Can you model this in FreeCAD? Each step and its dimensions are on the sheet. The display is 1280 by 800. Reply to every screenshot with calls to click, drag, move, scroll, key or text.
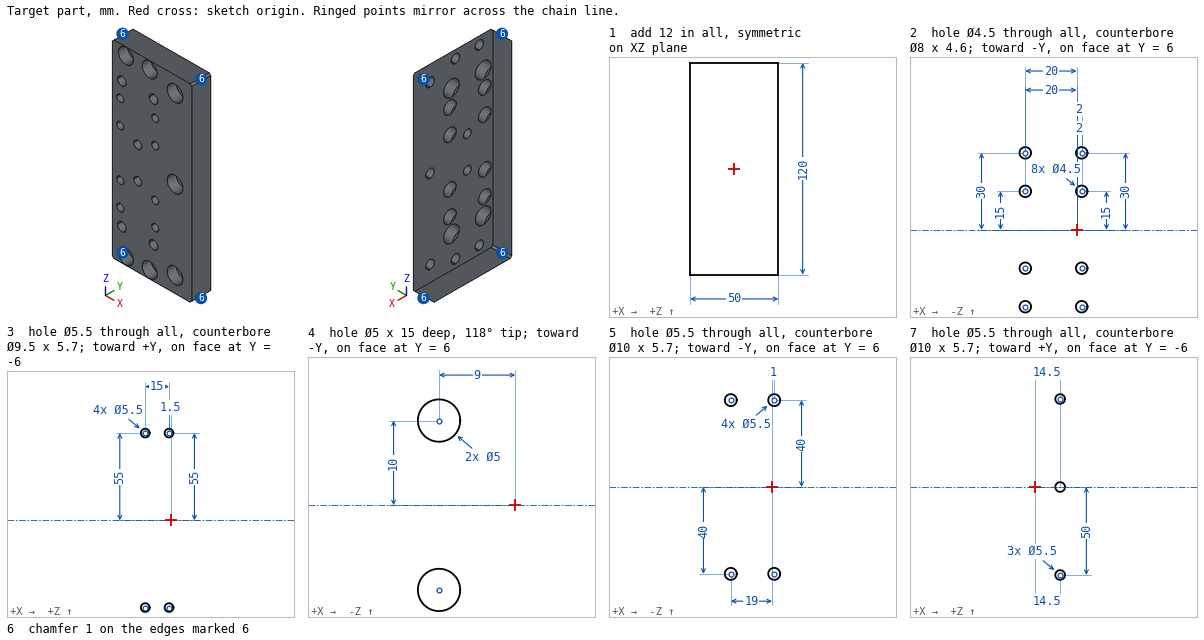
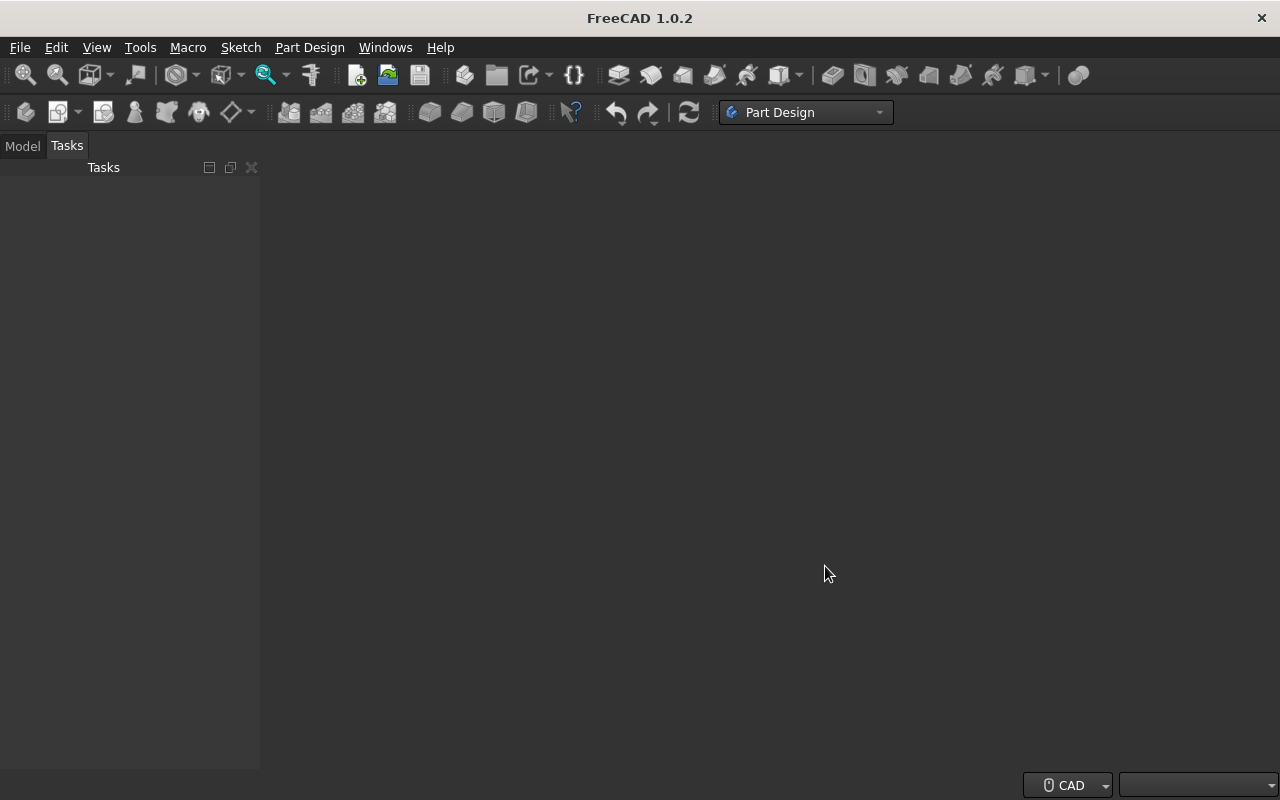
click(356, 76)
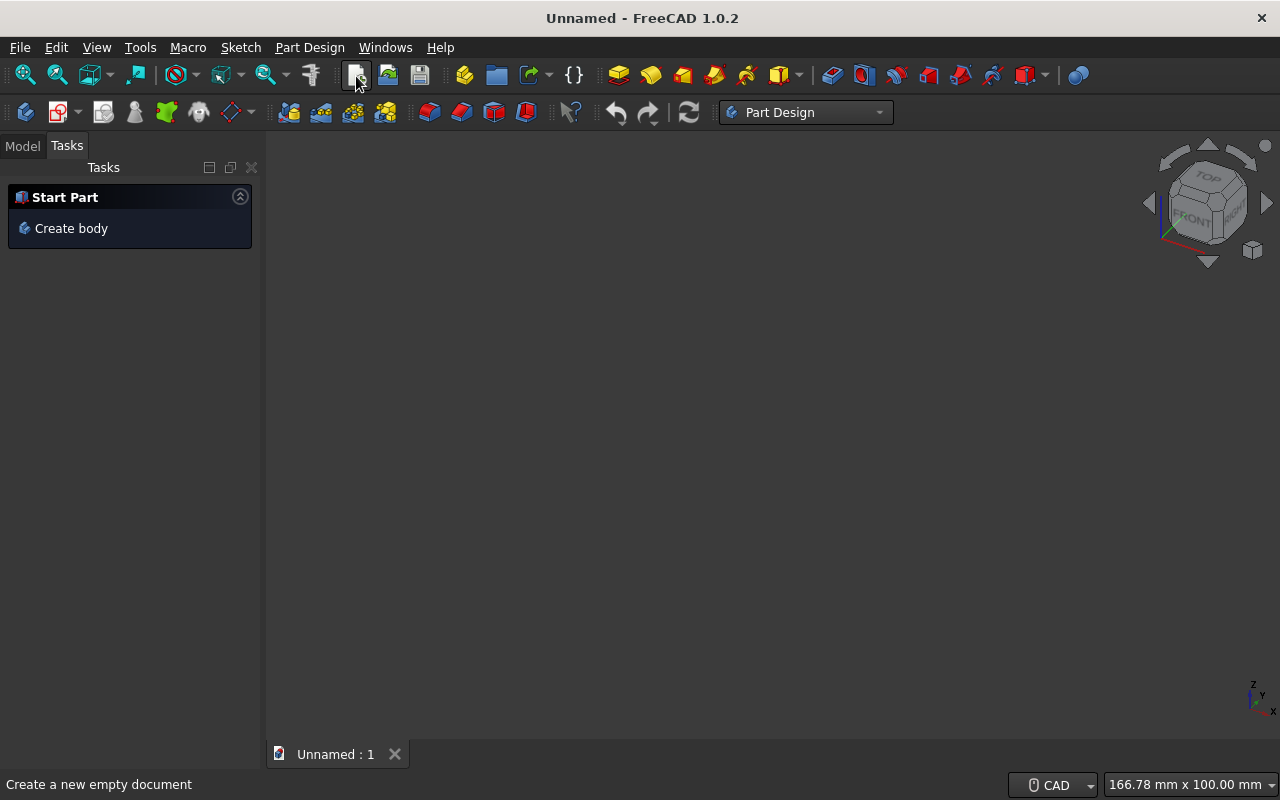
click(58, 112)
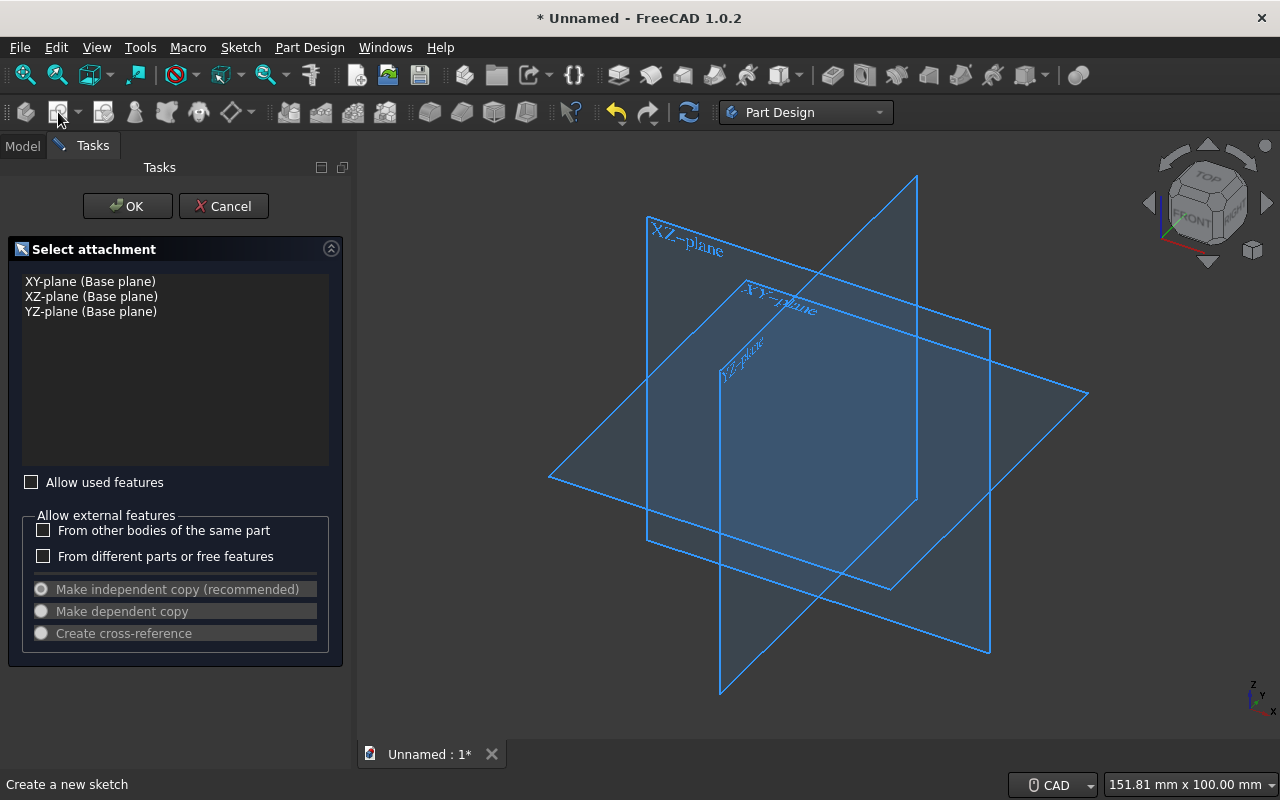
click(82, 296)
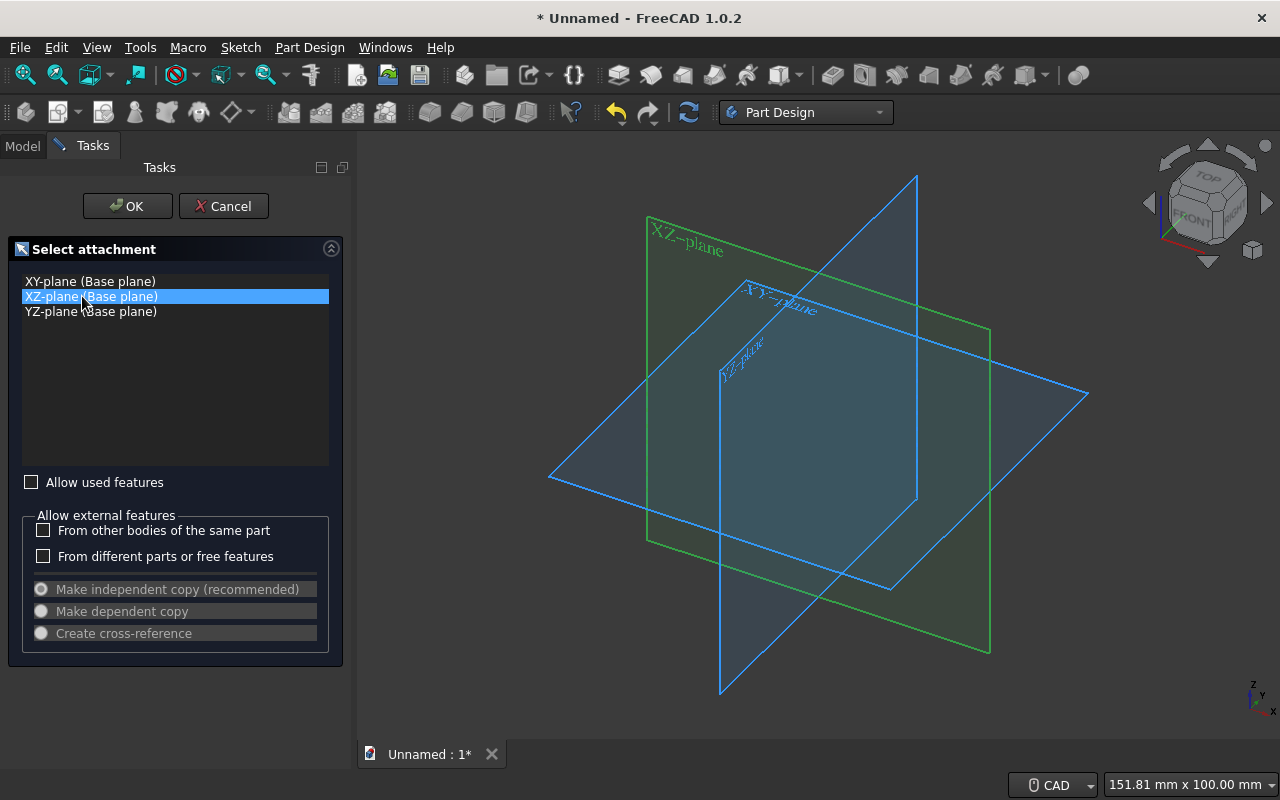
click(128, 206)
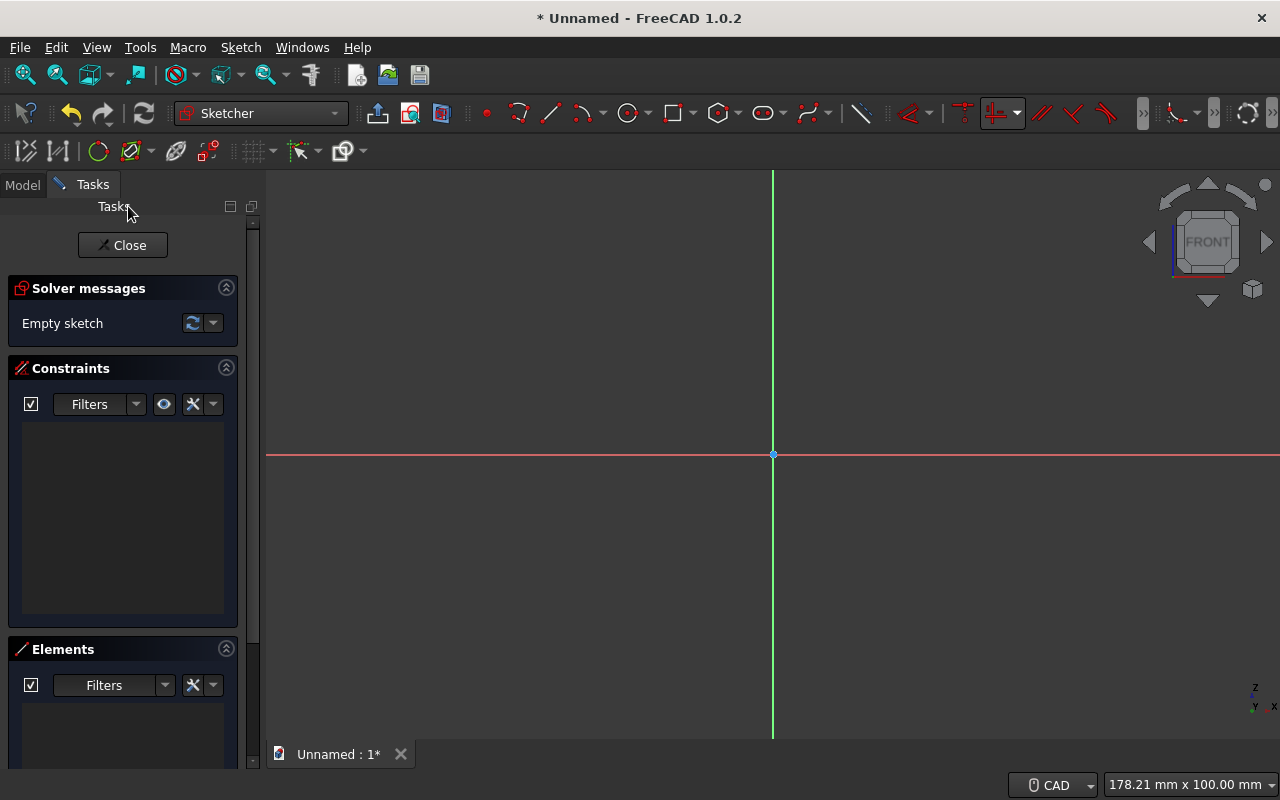
scroll(621, 454, down, 3)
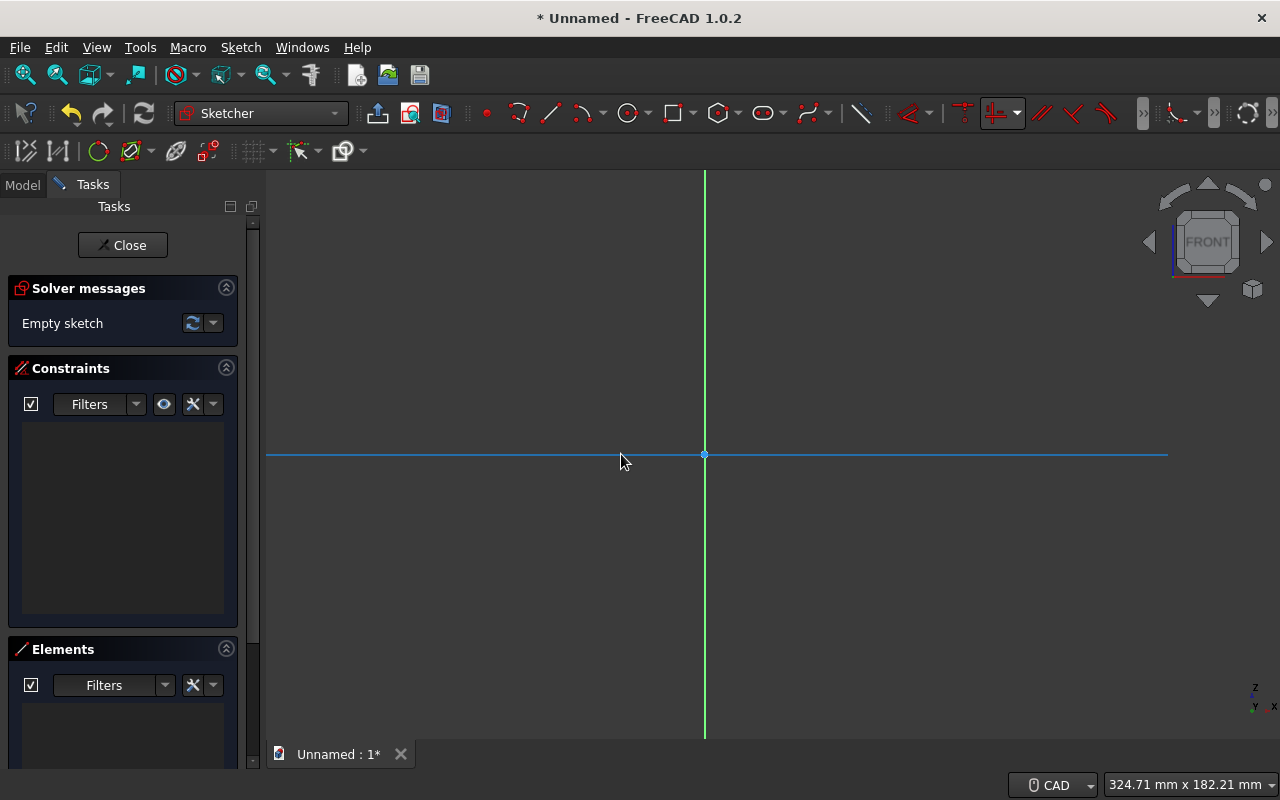
key(g)
key(v)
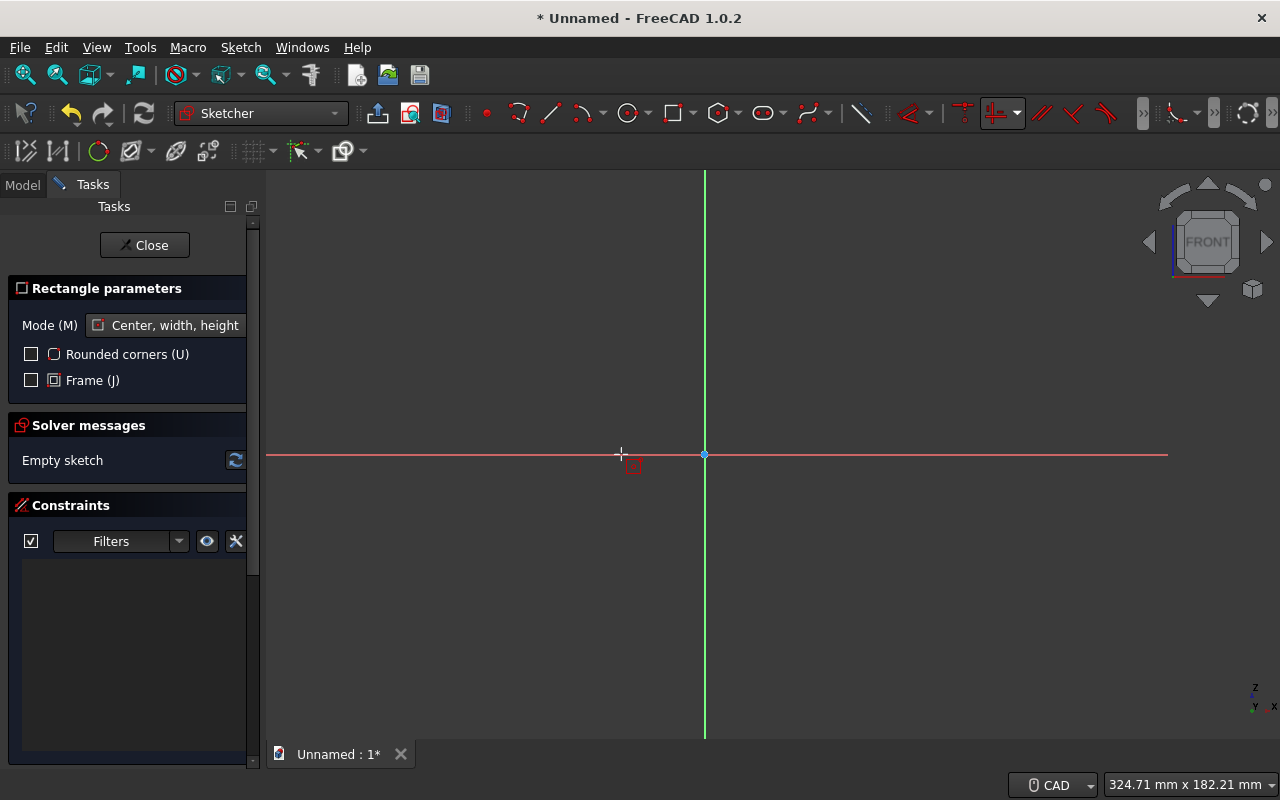
click(705, 454)
move(783, 267)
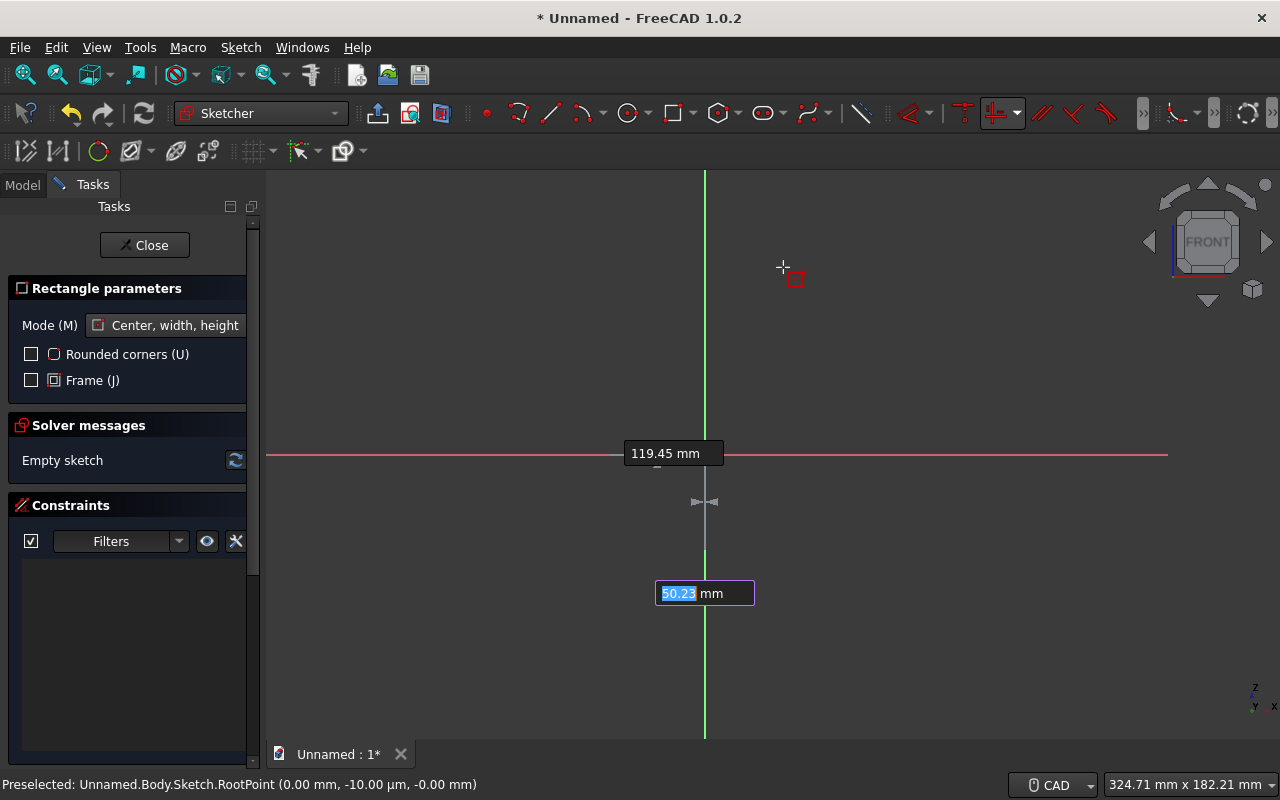
text(50)
key(Tab)
text(120)
key(Return)
key(Escape)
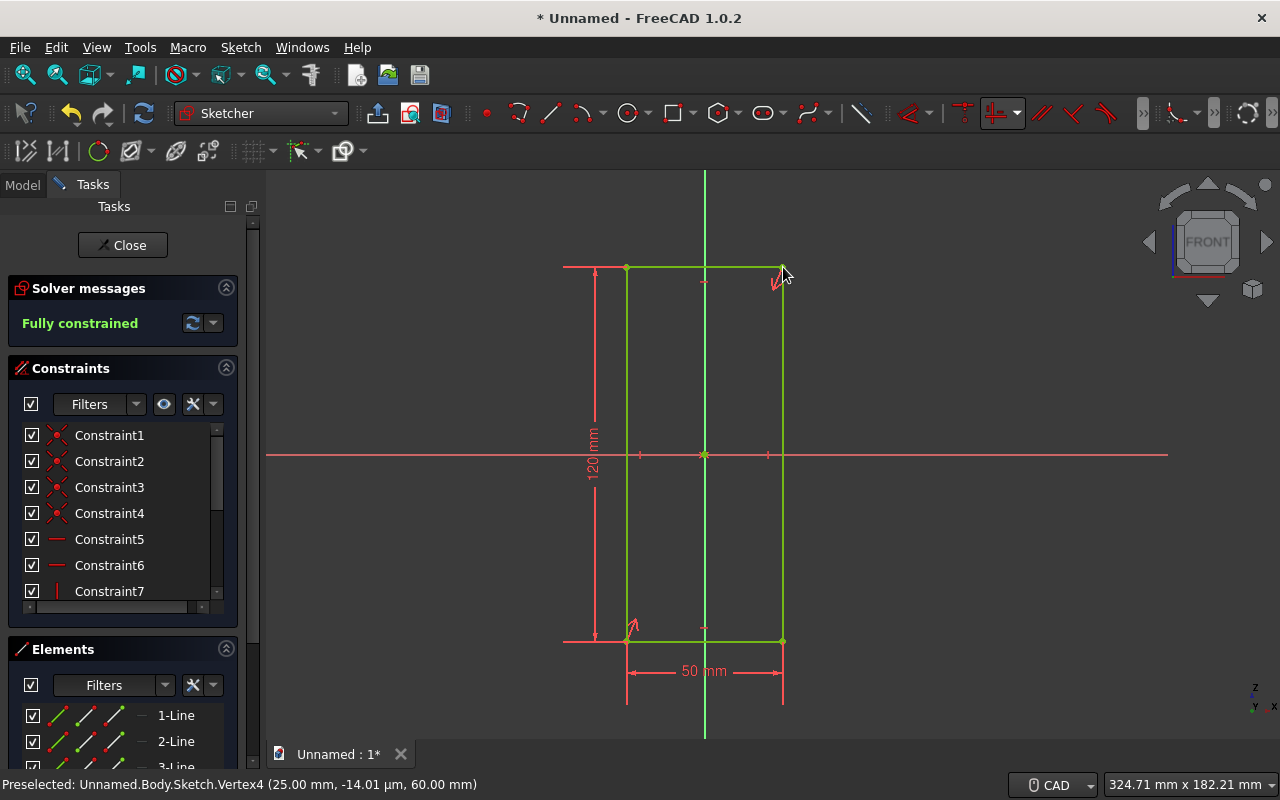
click(123, 245)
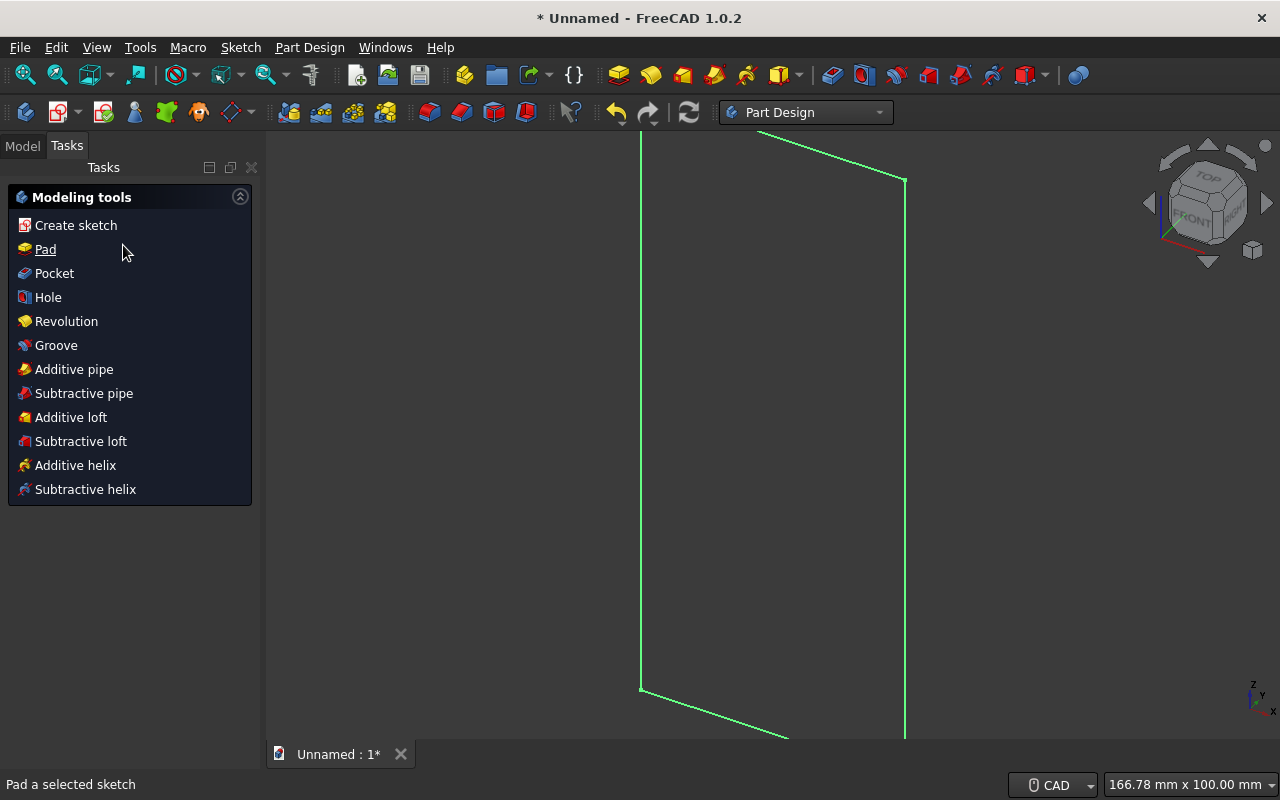
click(620, 76)